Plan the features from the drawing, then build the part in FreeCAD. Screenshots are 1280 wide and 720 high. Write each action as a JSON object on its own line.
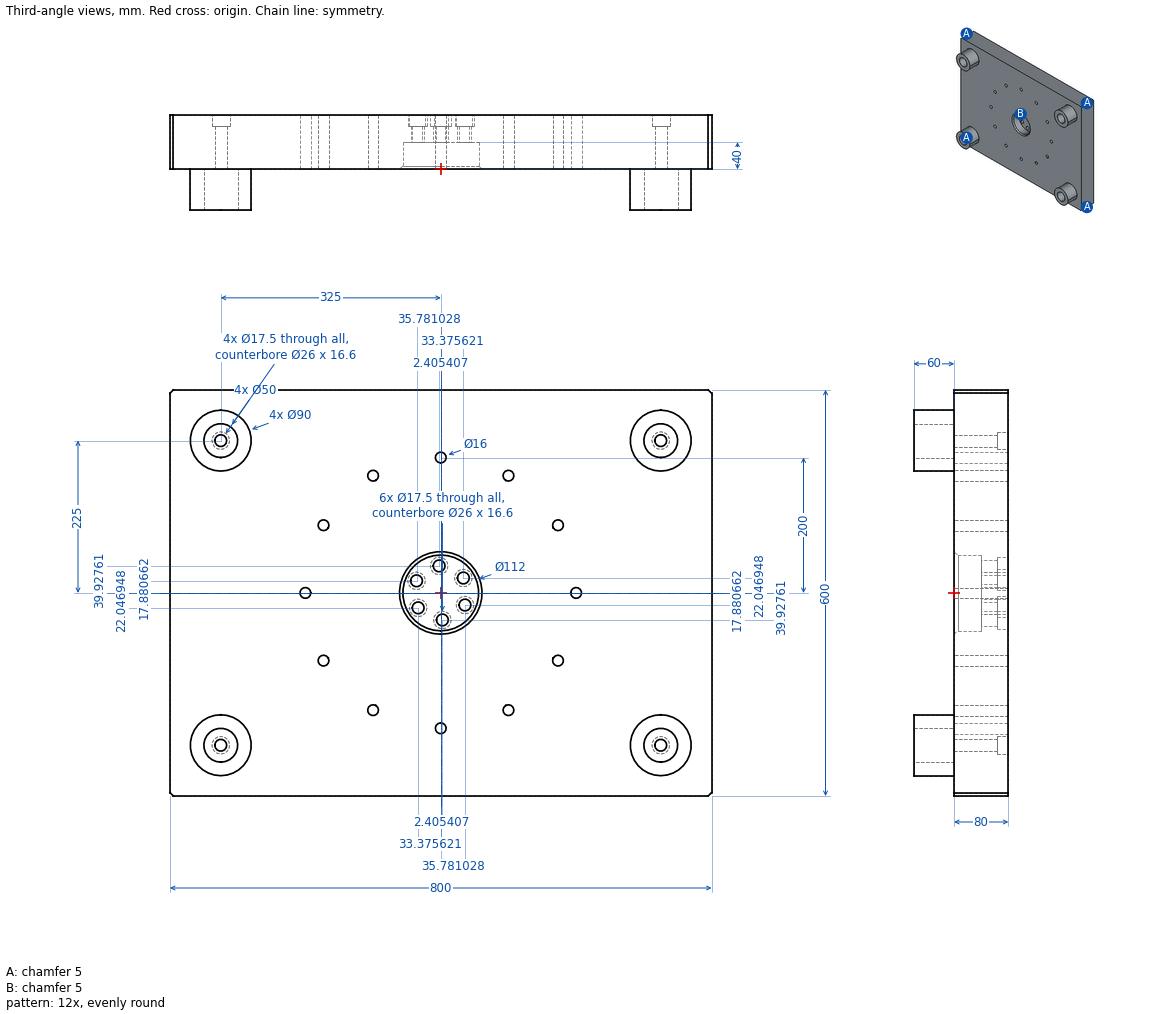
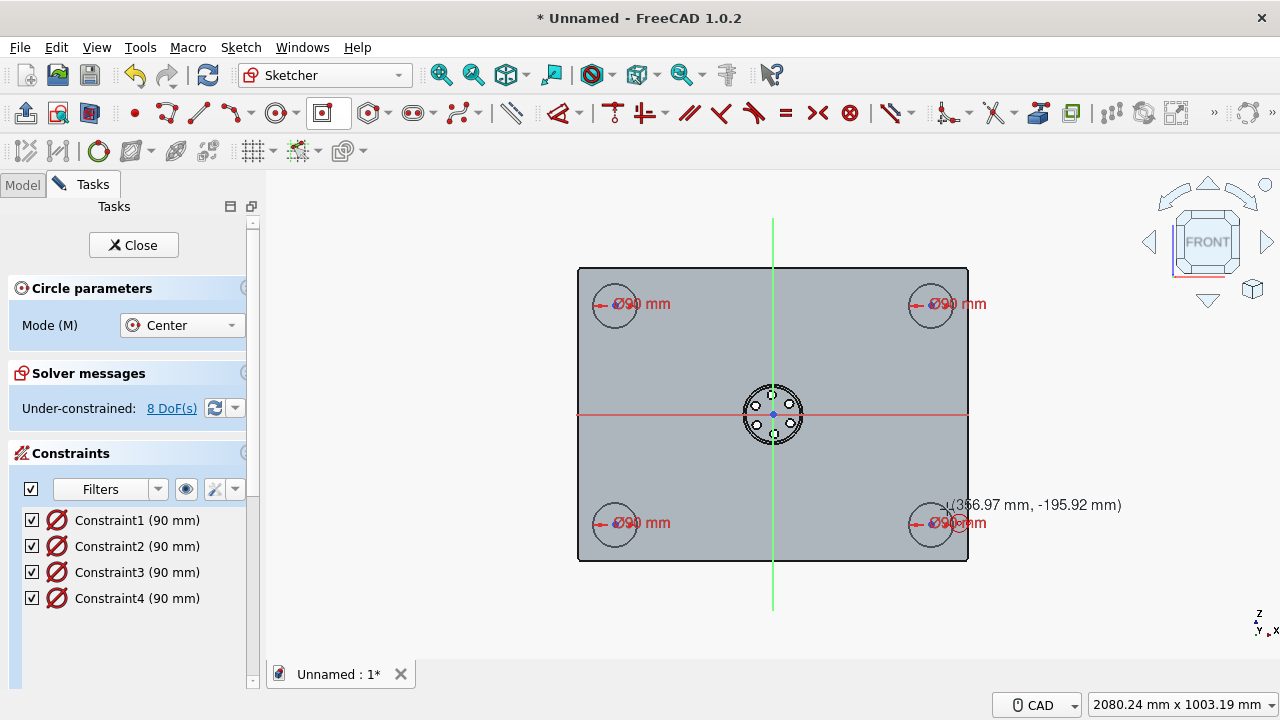
{"action": "scroll", "coordinate": [615, 305], "scroll_direction": "up", "scroll_amount": 4}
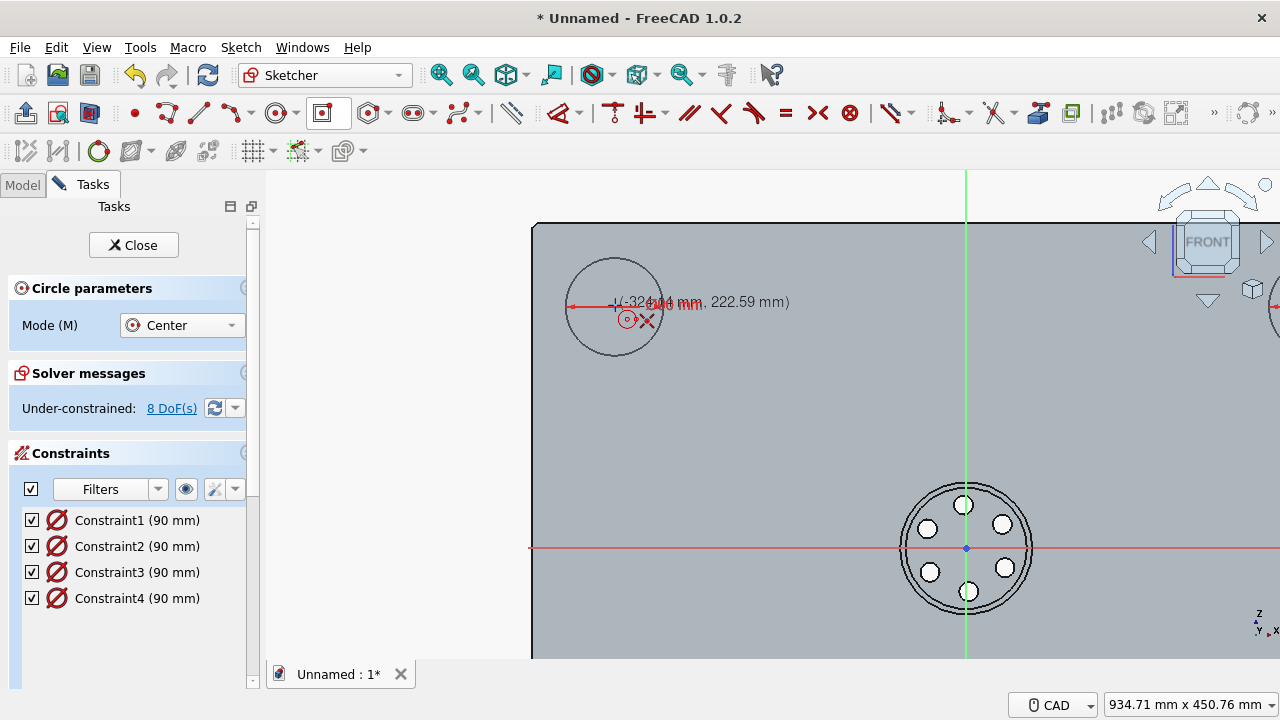
{"action": "left_click", "coordinate": [615, 307]}
{"action": "mouse_move", "coordinate": [633, 285]}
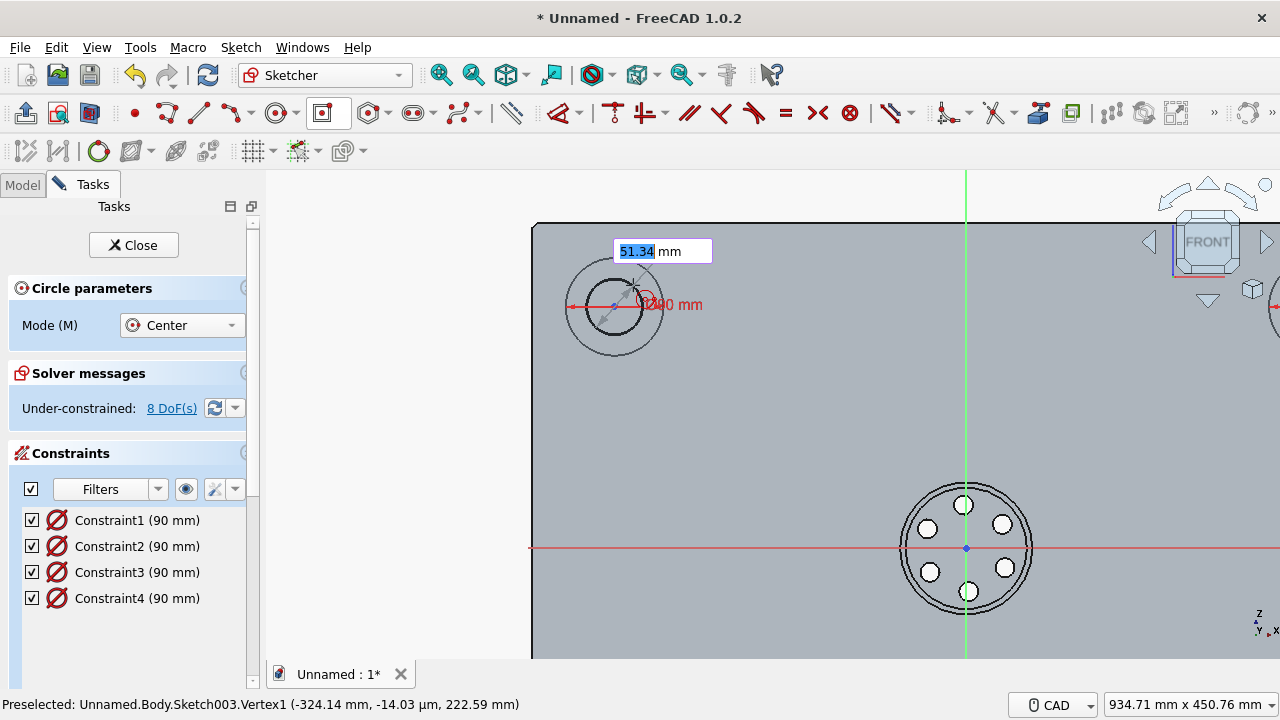
{"action": "type", "text": "50"}
{"action": "key", "text": "Return"}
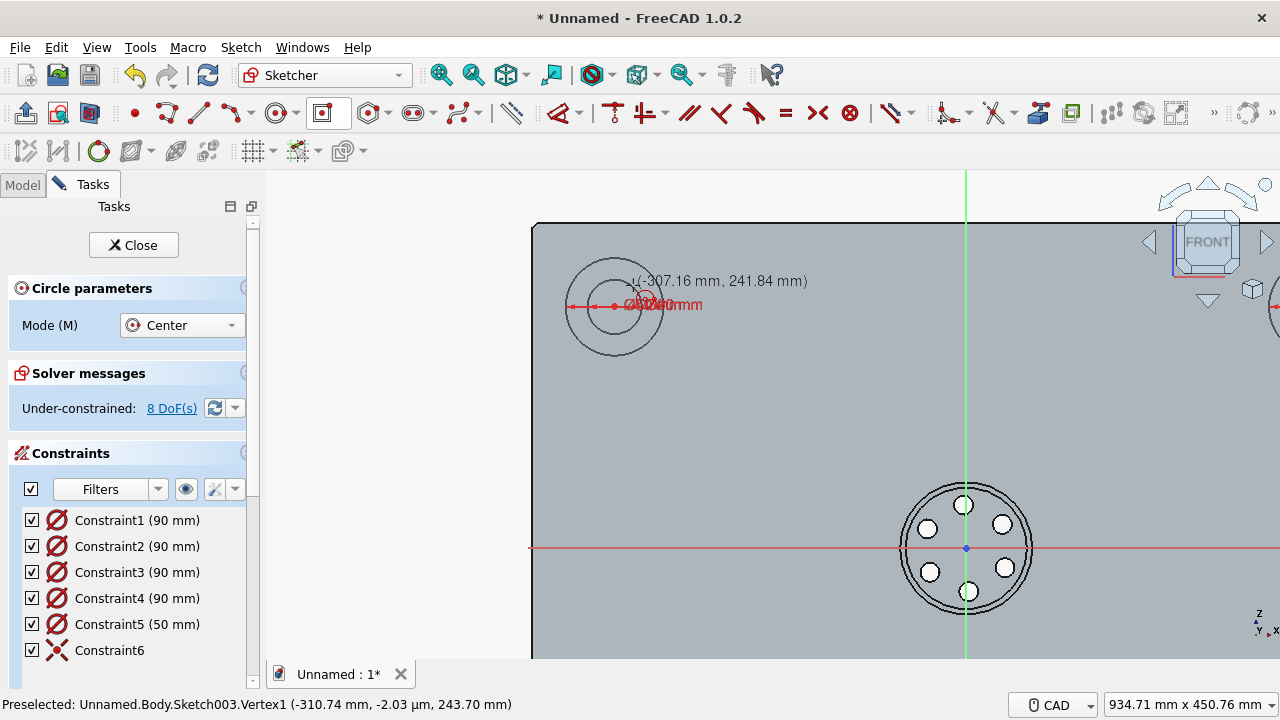
{"action": "scroll", "coordinate": [386, 252], "scroll_direction": "down", "scroll_amount": 3}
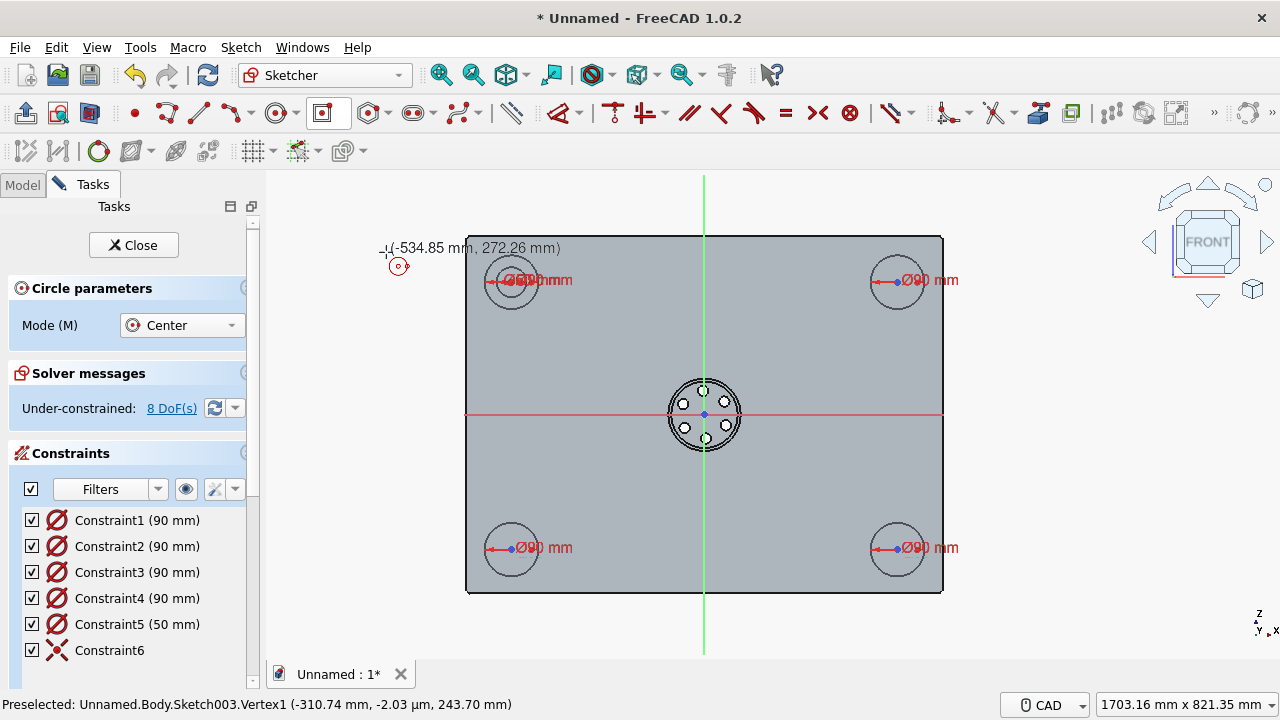
{"action": "scroll", "coordinate": [898, 281], "scroll_direction": "up", "scroll_amount": 3}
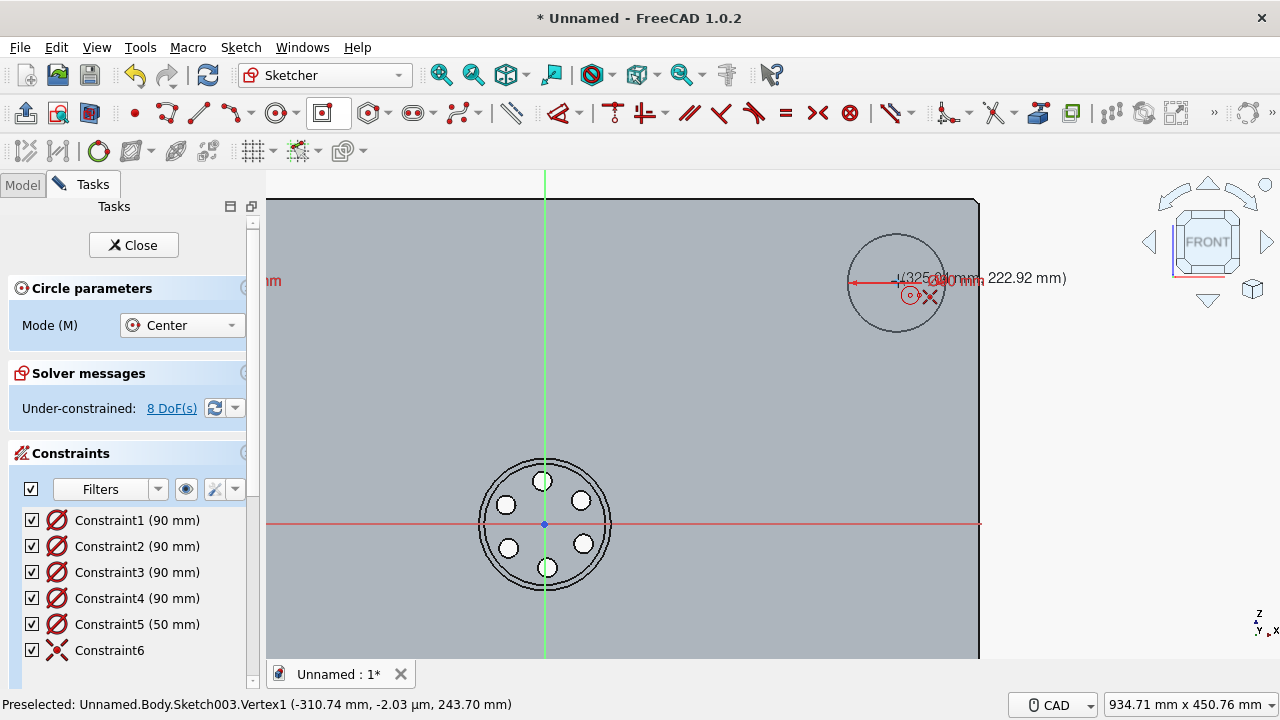
{"action": "left_click", "coordinate": [897, 283]}
{"action": "mouse_move", "coordinate": [917, 261]}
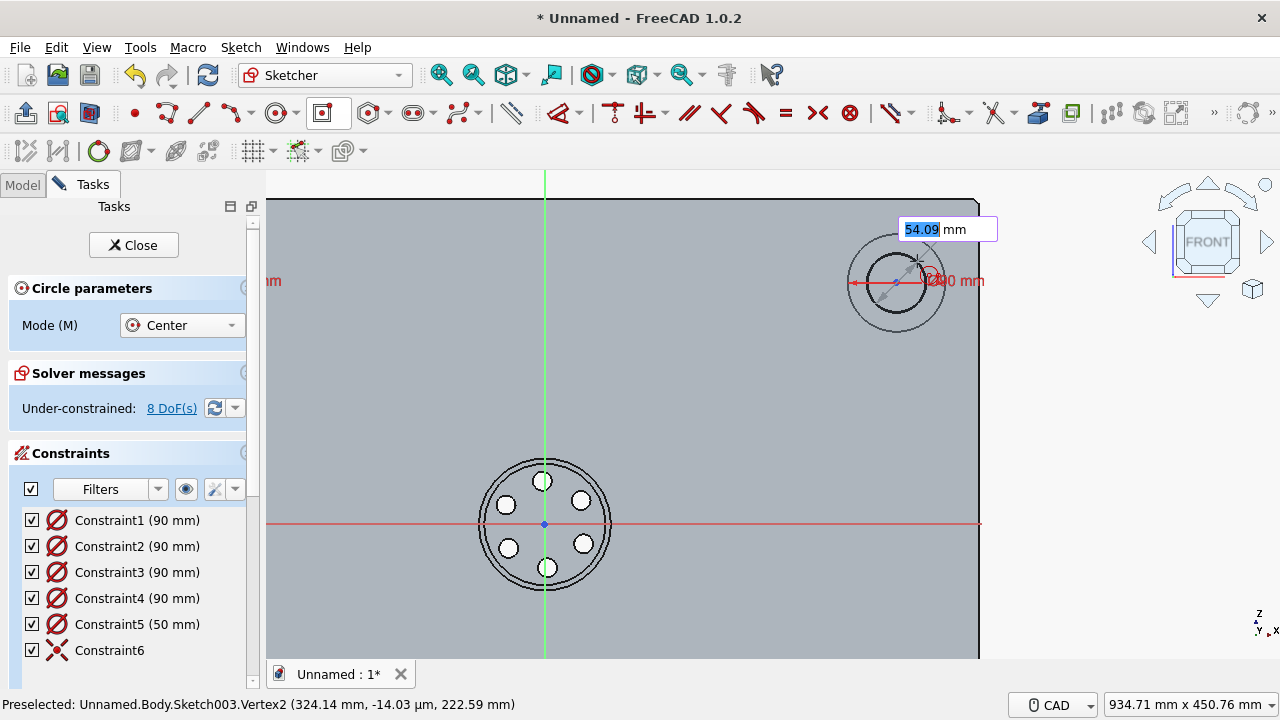
{"action": "type", "text": "50"}
{"action": "key", "text": "Return"}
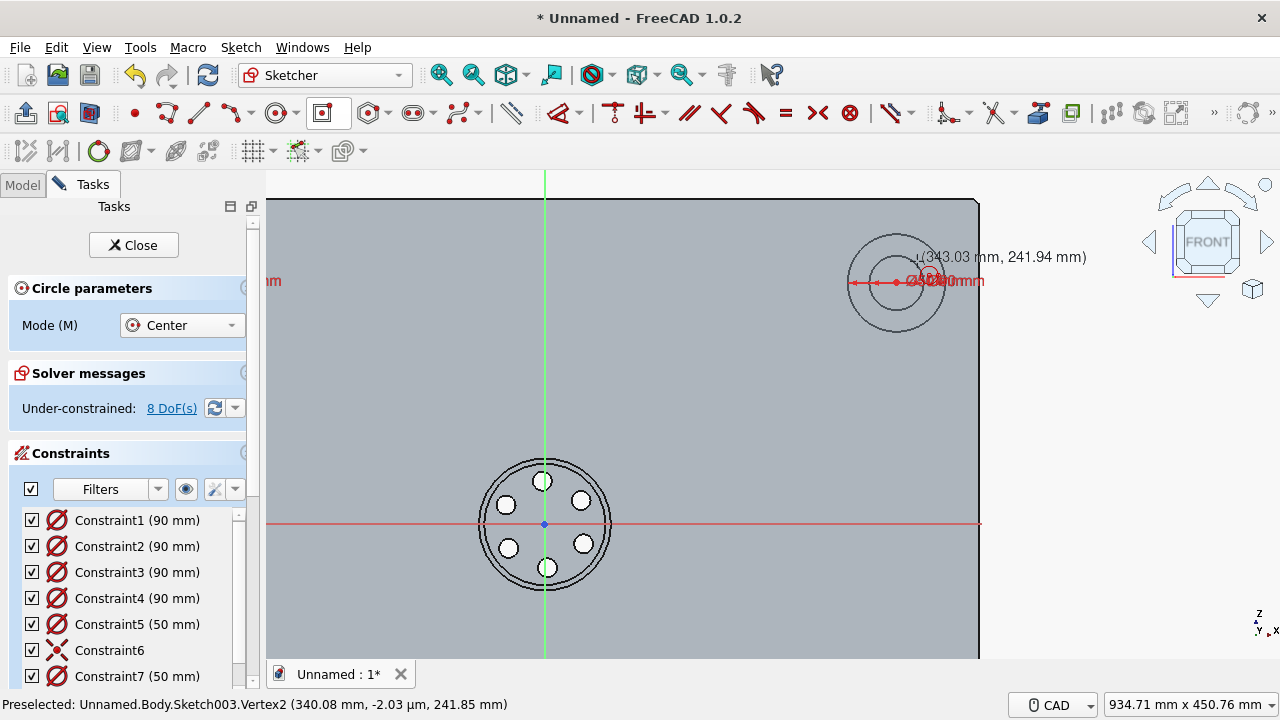
{"action": "scroll", "coordinate": [899, 281], "scroll_direction": "down", "scroll_amount": 3}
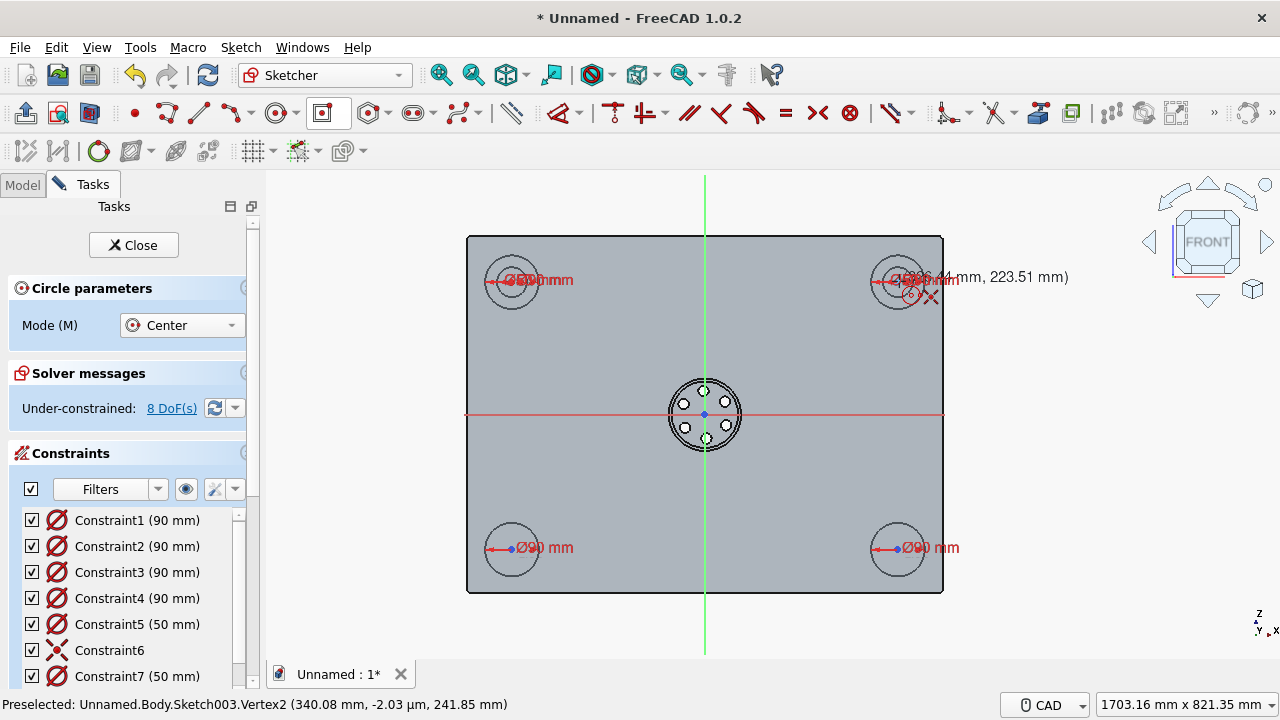
{"action": "scroll", "coordinate": [511, 549], "scroll_direction": "up", "scroll_amount": 3}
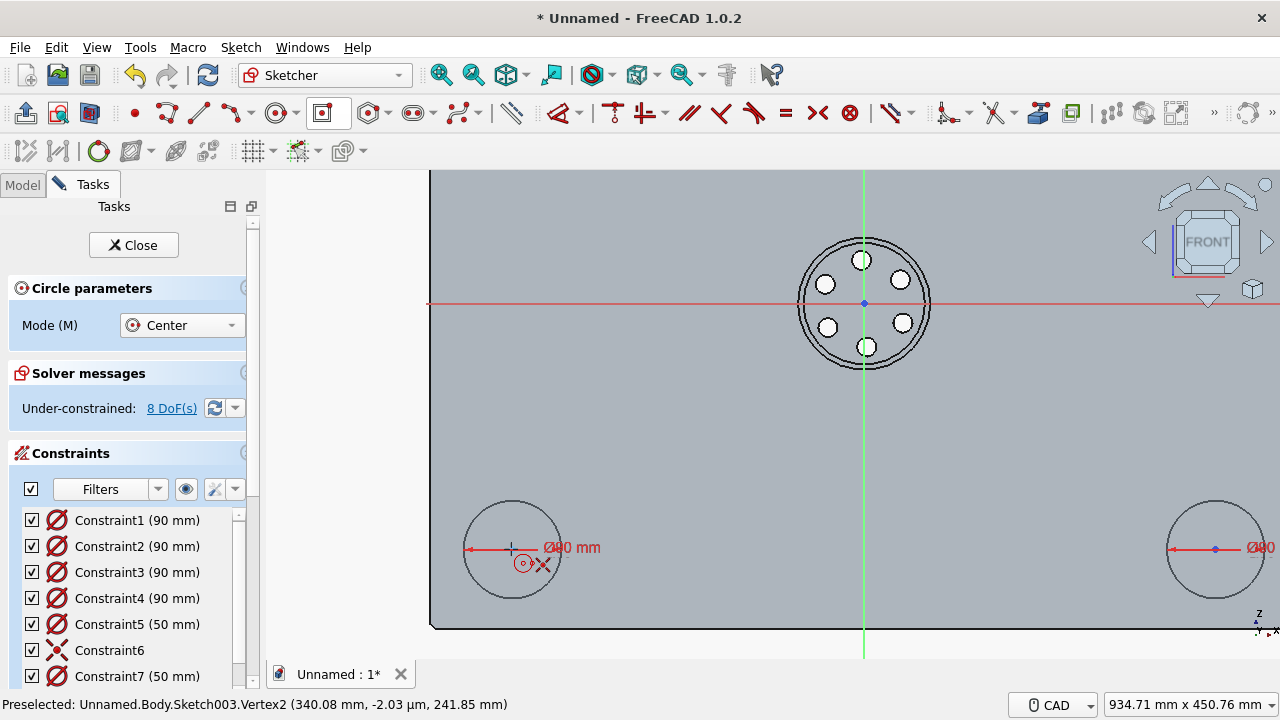
{"action": "left_click", "coordinate": [513, 550]}
{"action": "mouse_move", "coordinate": [531, 529]}